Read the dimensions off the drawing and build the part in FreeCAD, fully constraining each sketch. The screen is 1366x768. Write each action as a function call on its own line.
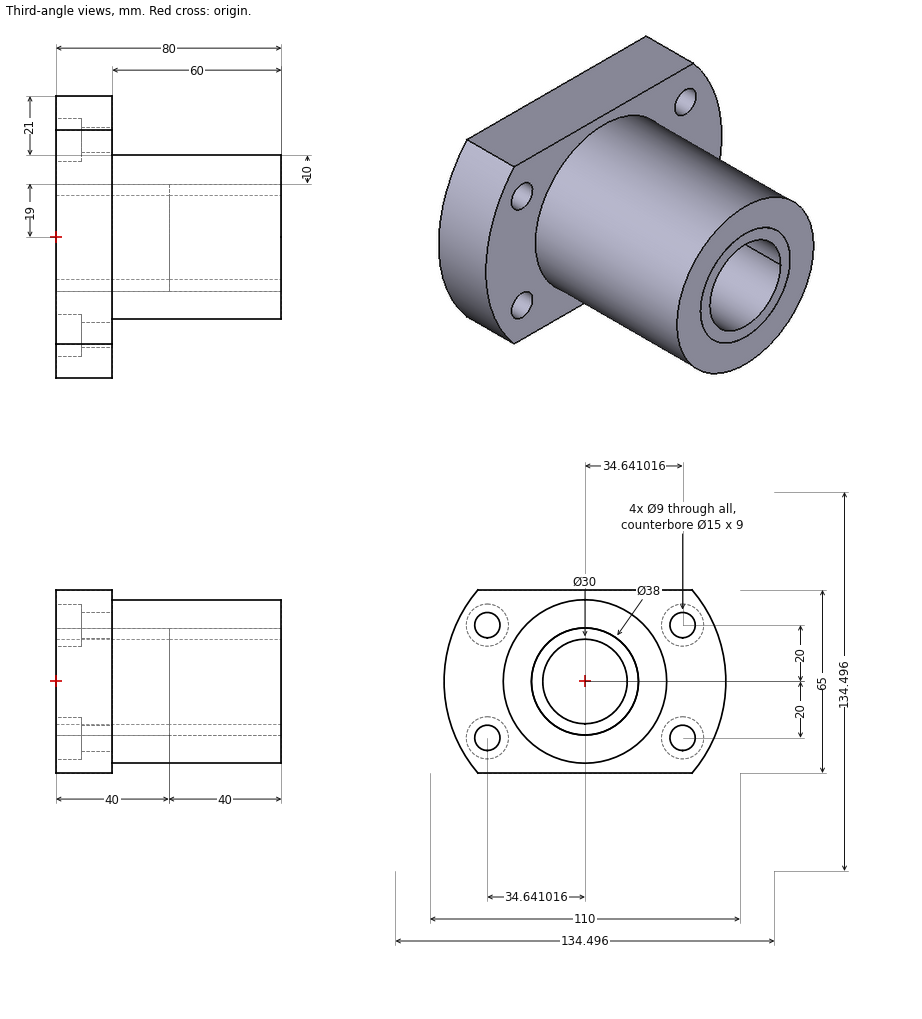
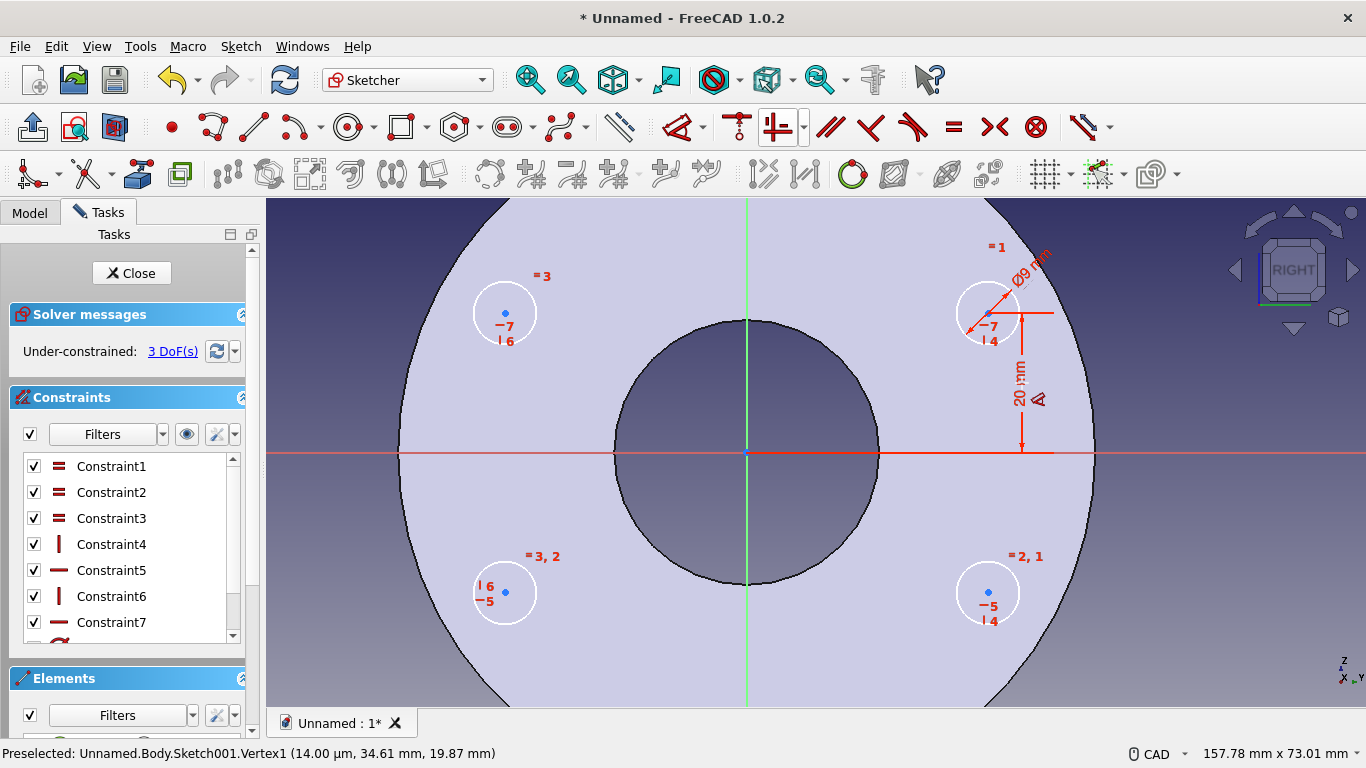
click(988, 593)
click(1022, 523)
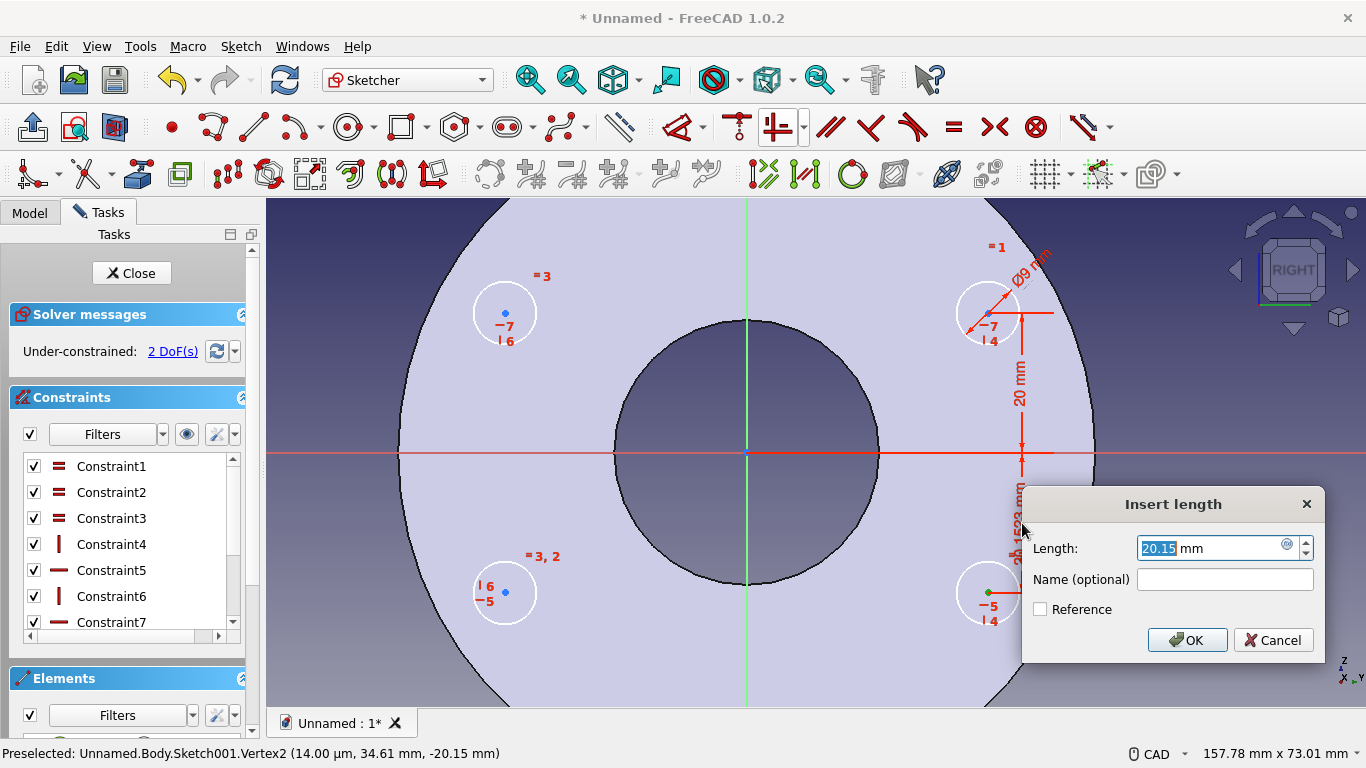
text(20)
key(Return)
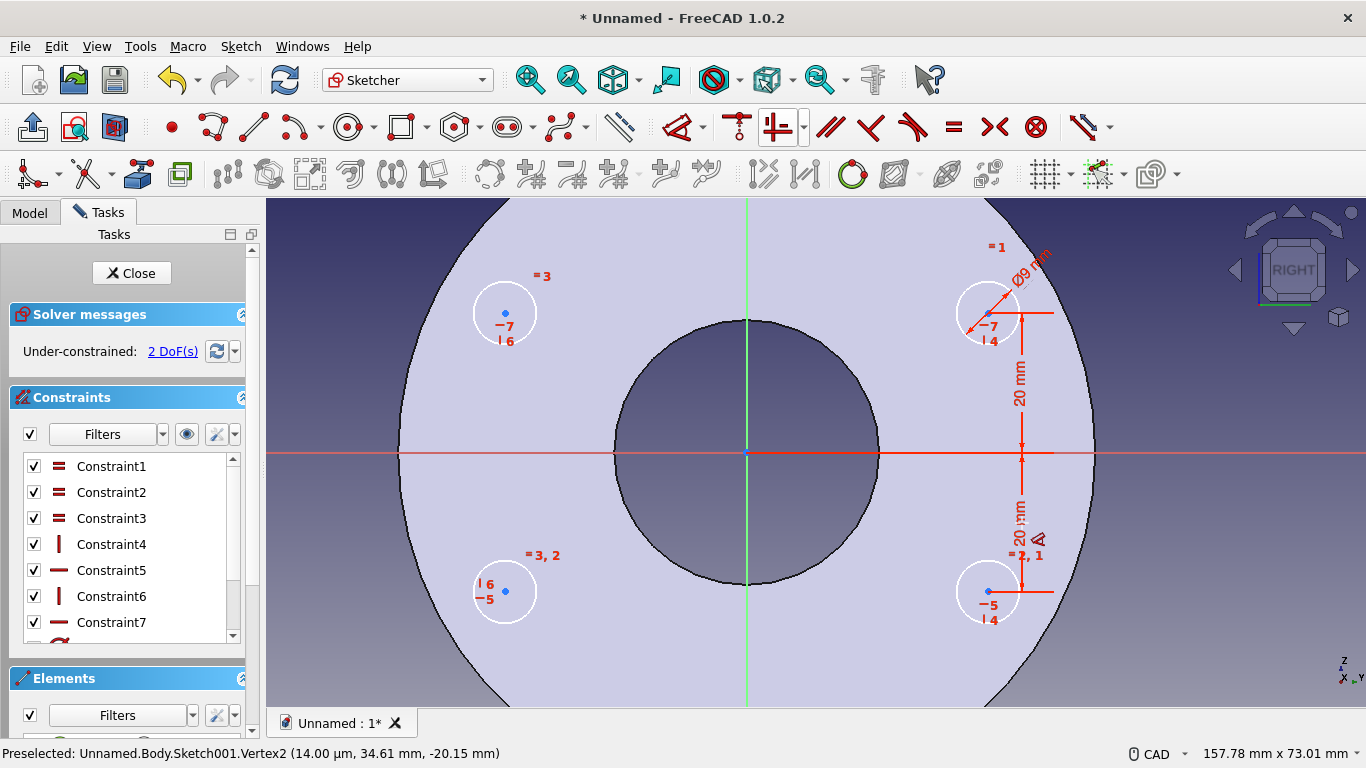
click(988, 313)
click(867, 279)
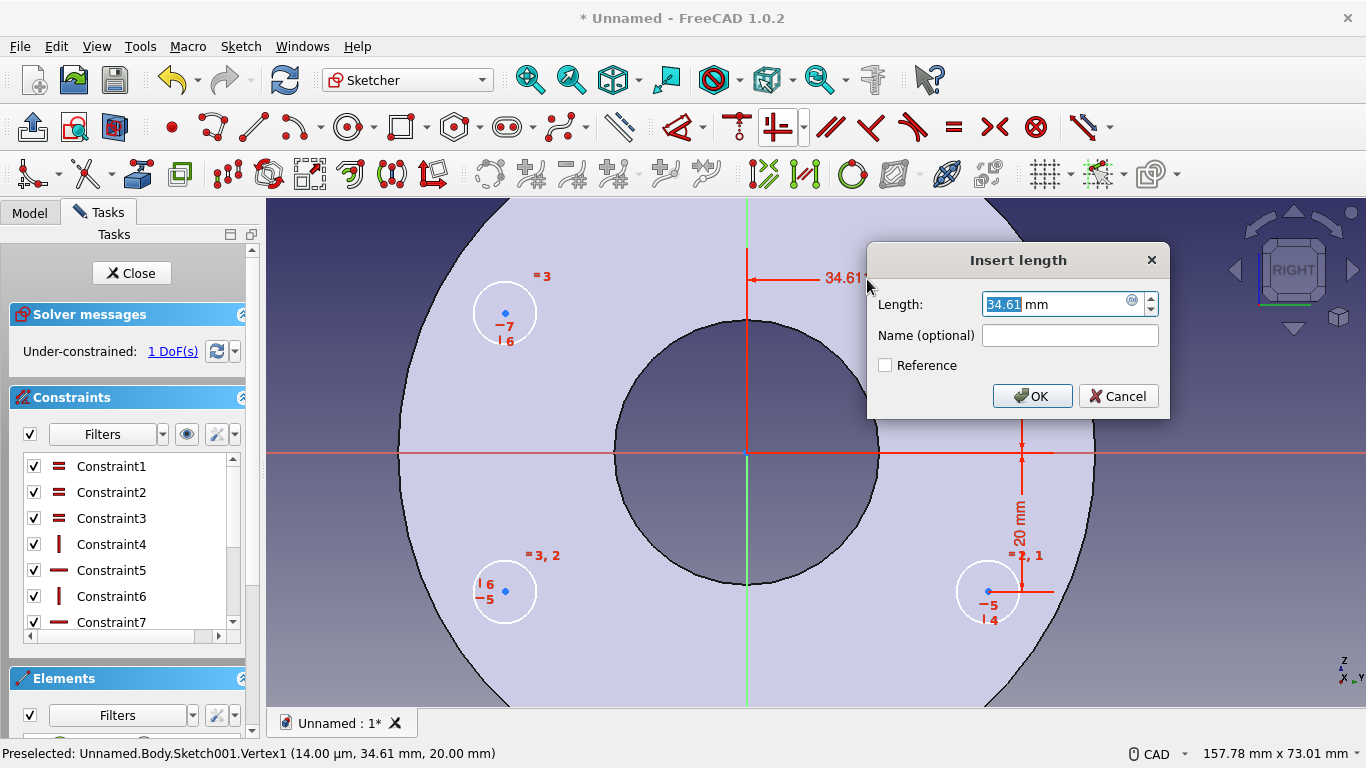
text(34.641016)
key(Return)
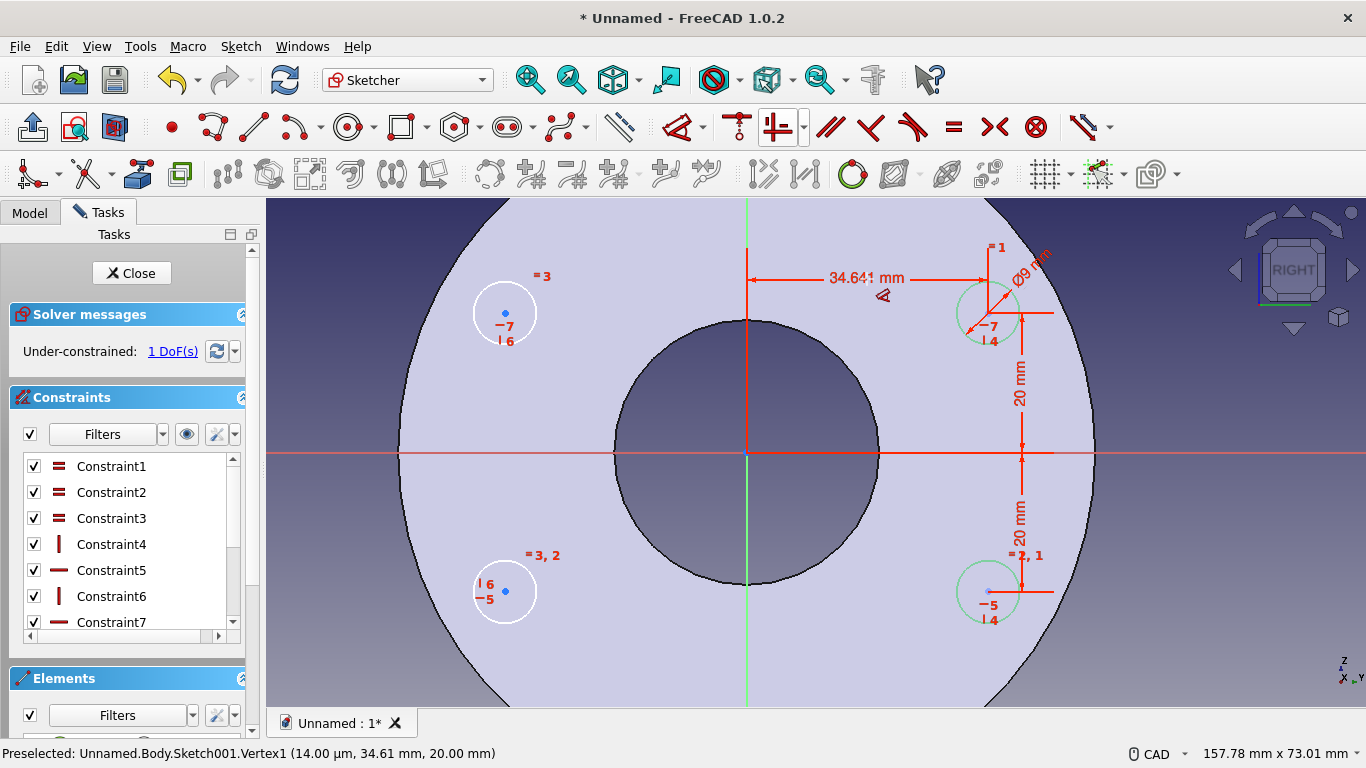
click(505, 592)
click(626, 626)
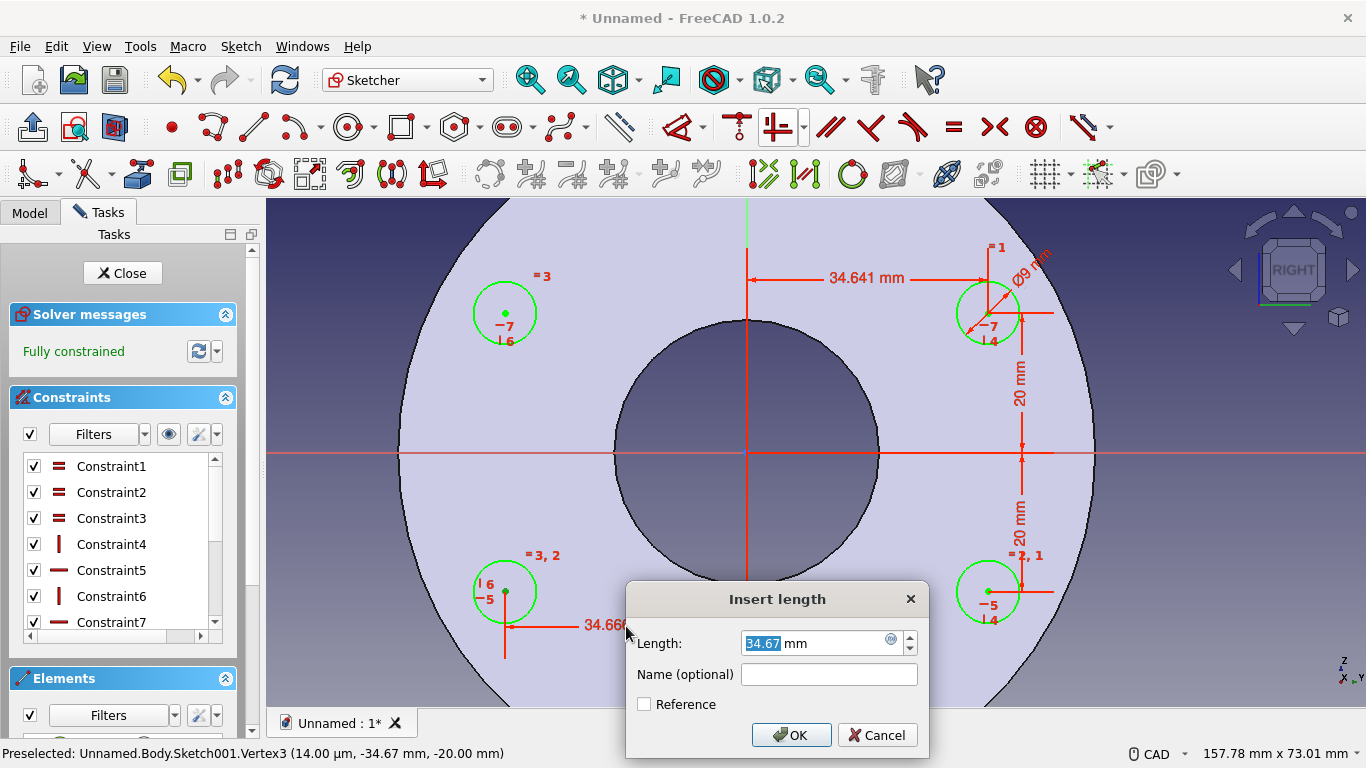
text(34.641016)
key(Return)
key(Escape)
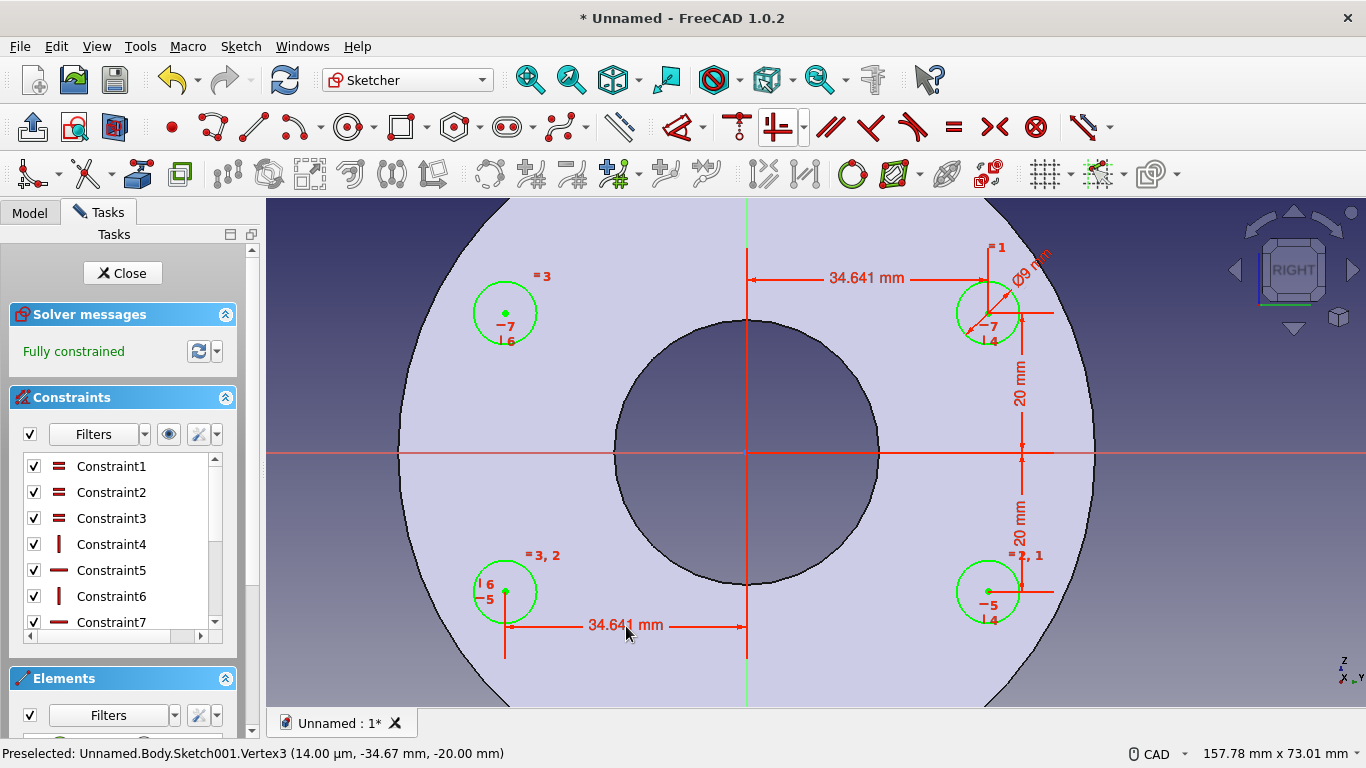
click(123, 273)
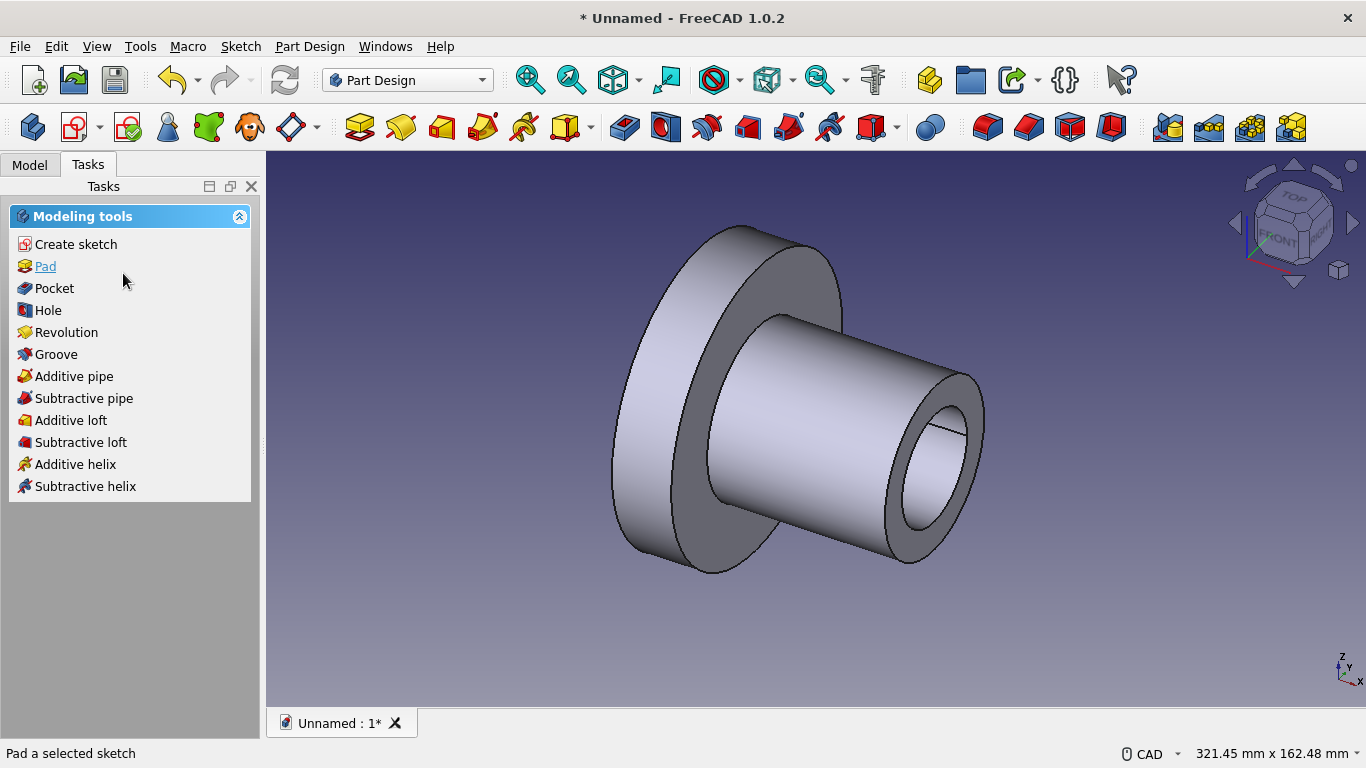
click(666, 128)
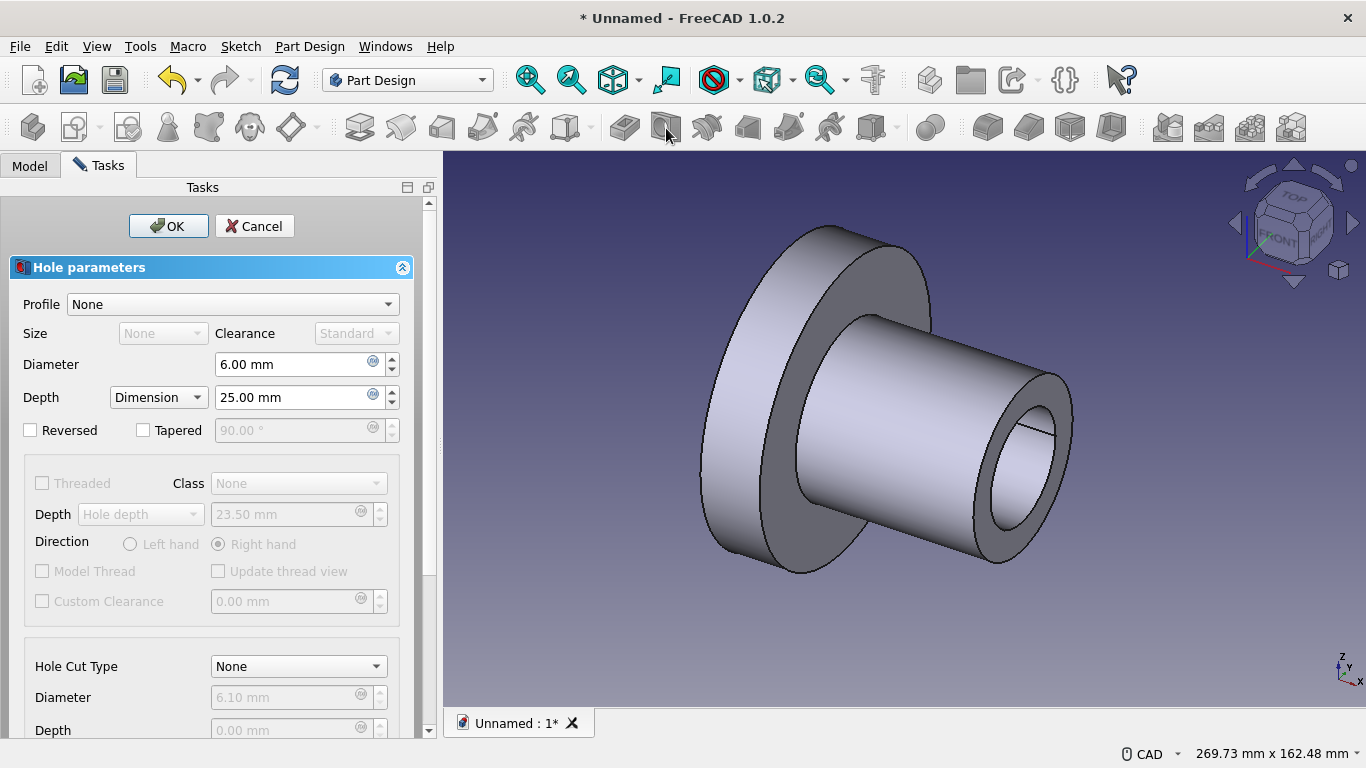
triple_click(300, 364)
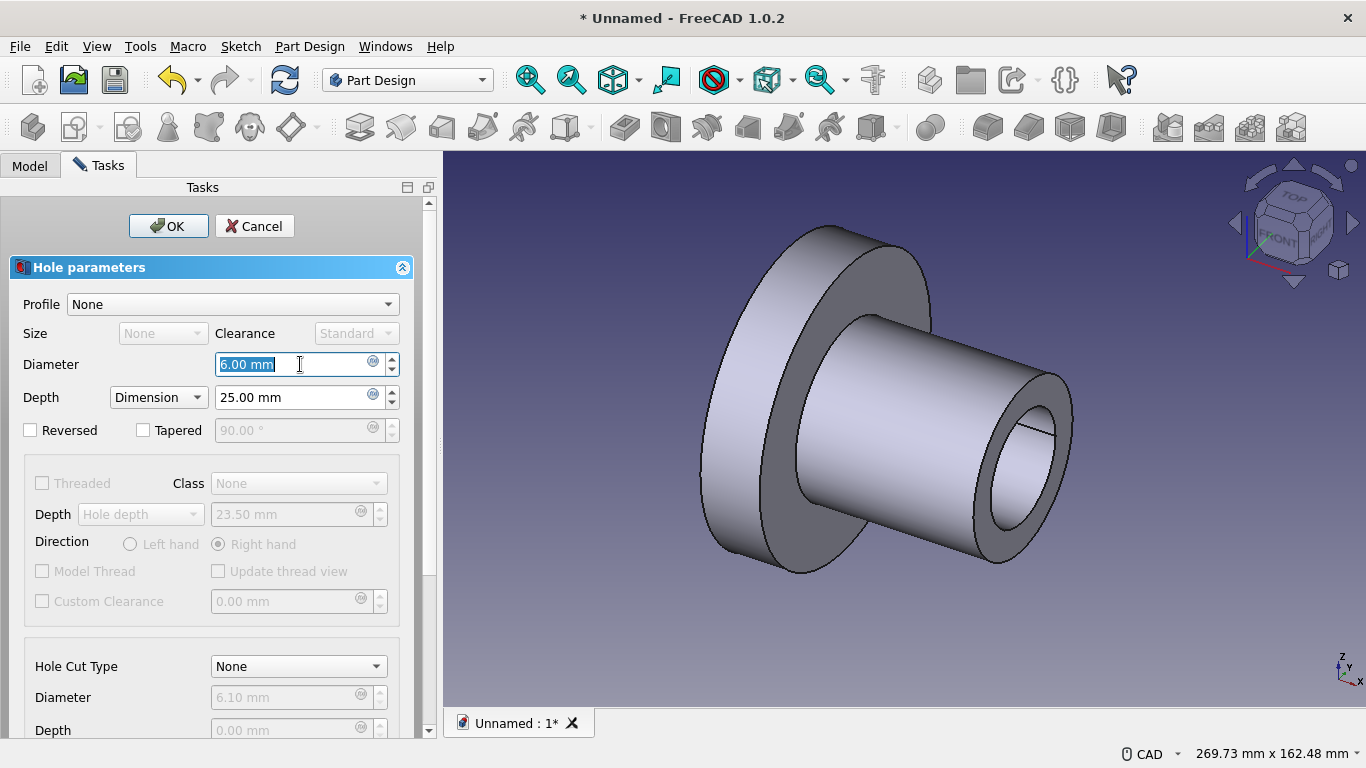
text(9)
key(Tab)